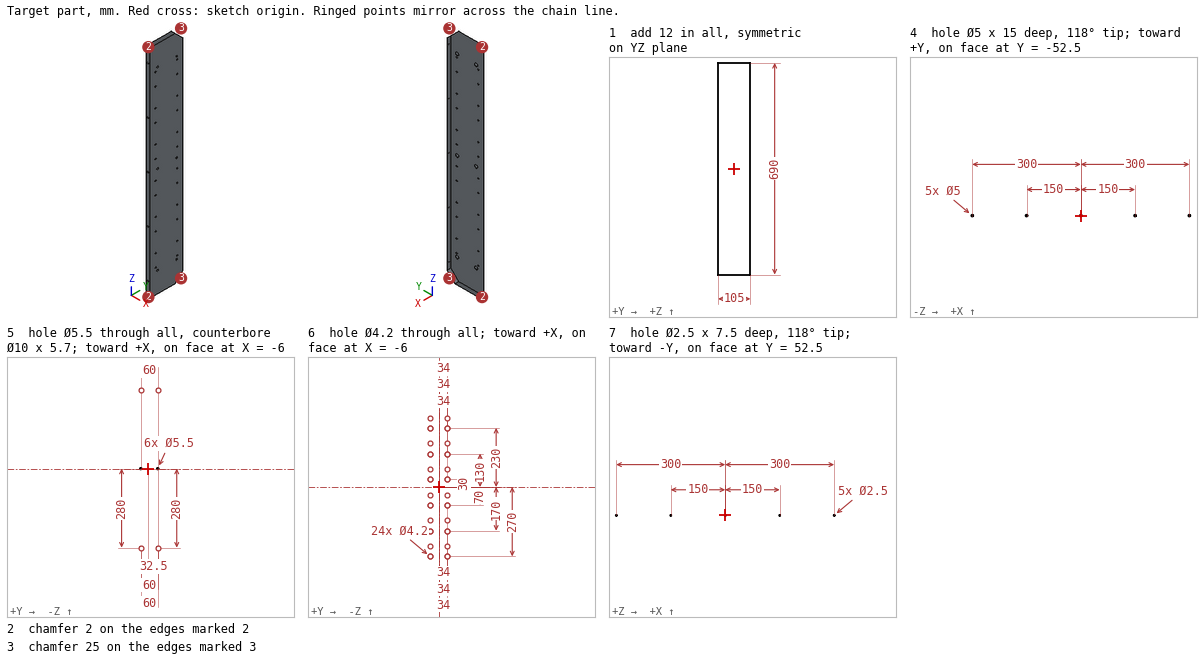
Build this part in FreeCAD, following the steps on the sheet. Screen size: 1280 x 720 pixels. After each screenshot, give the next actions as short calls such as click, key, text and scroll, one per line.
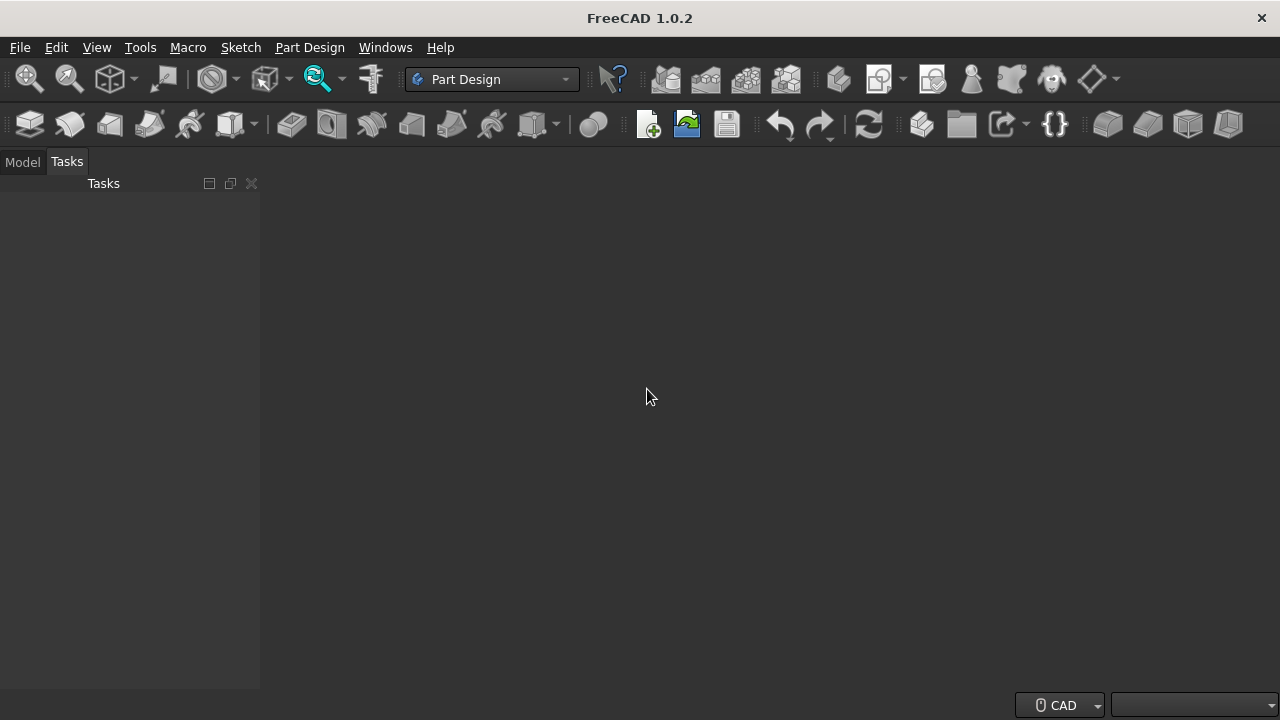
key(ctrl+n)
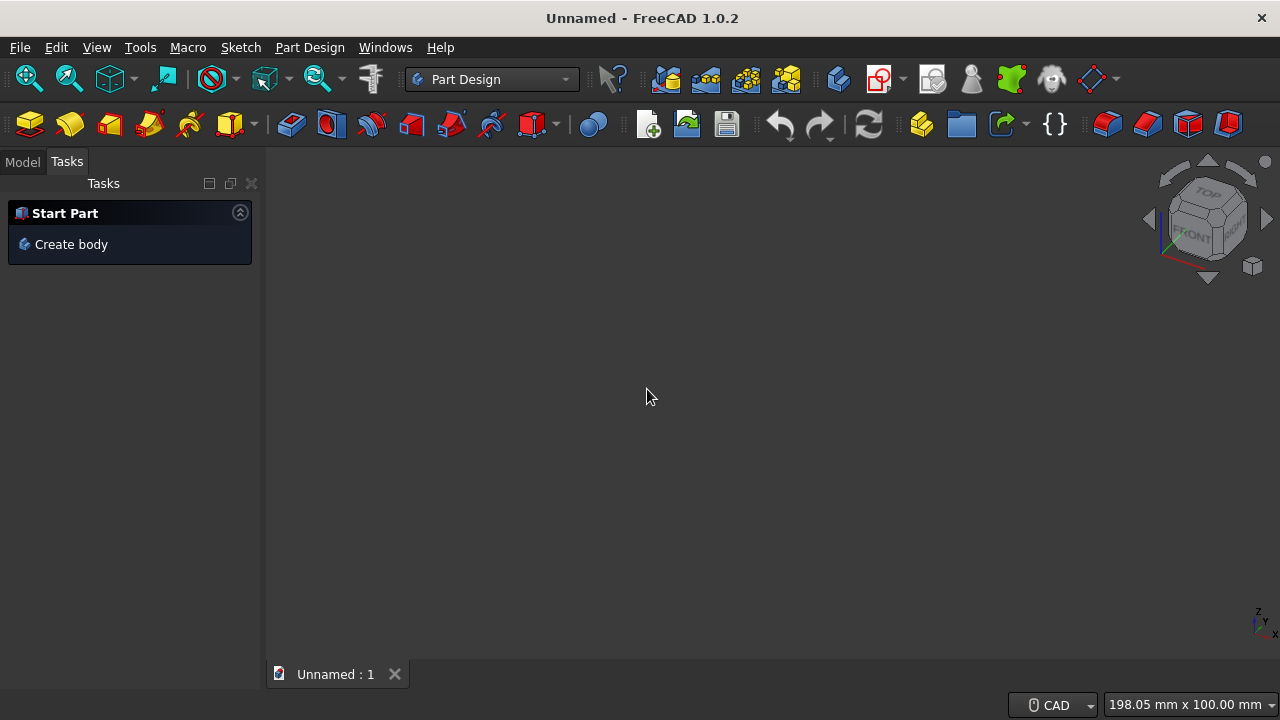
click(880, 80)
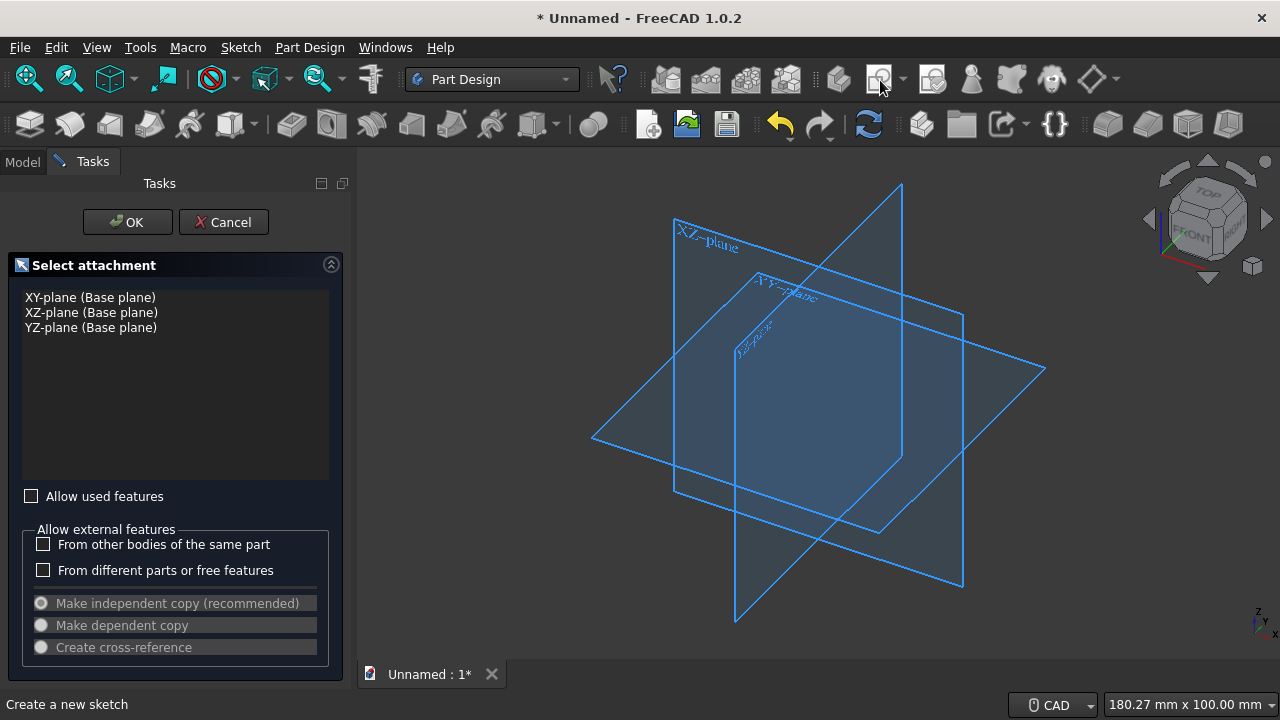
click(82, 328)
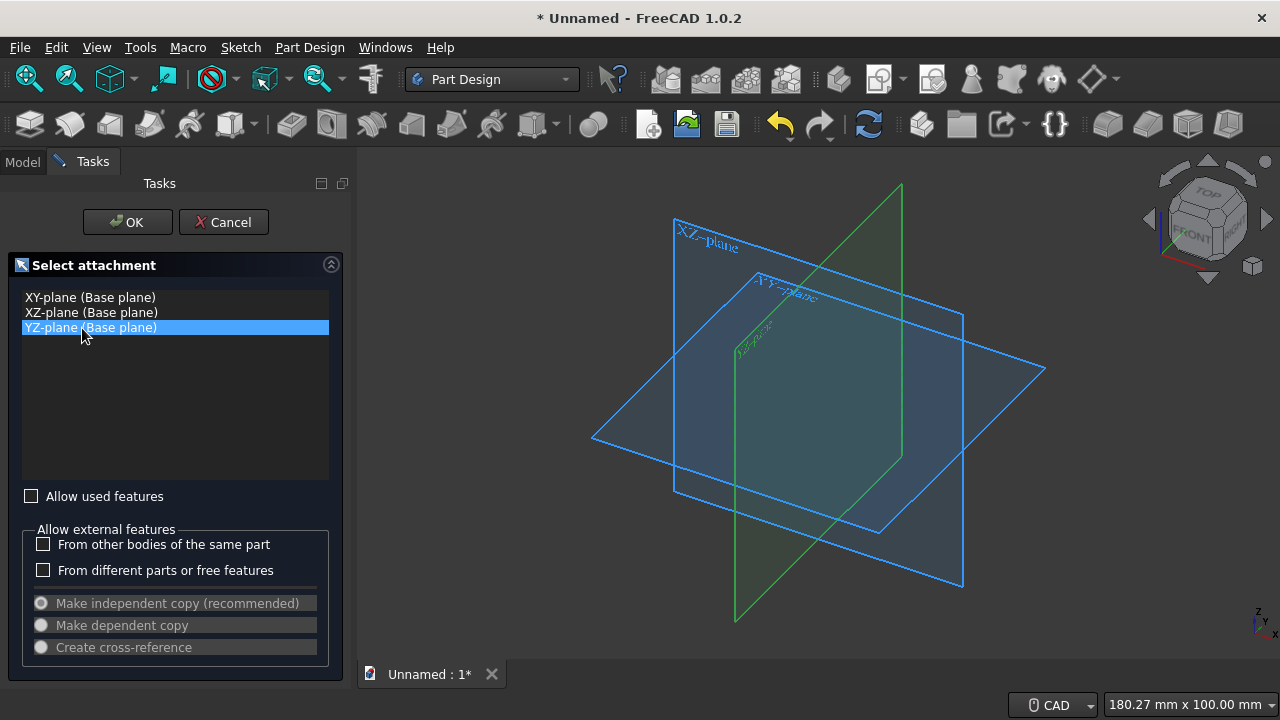
click(128, 222)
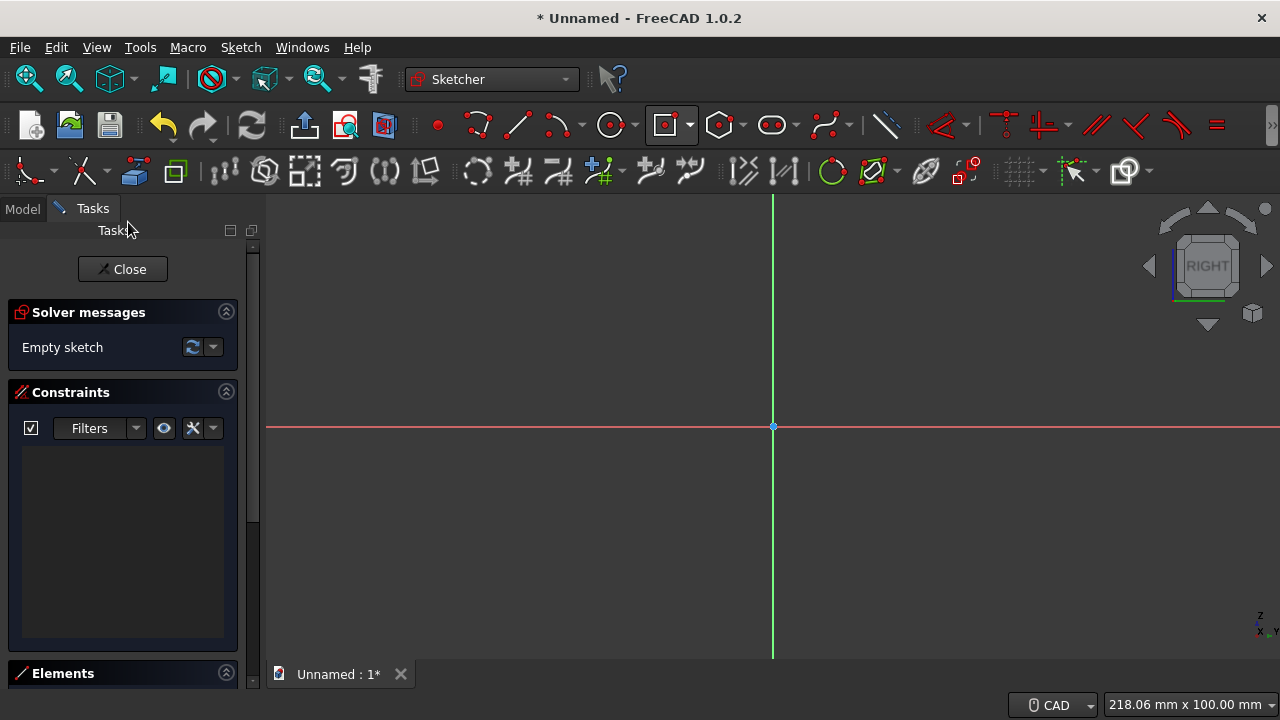
scroll(698, 426, down, 12)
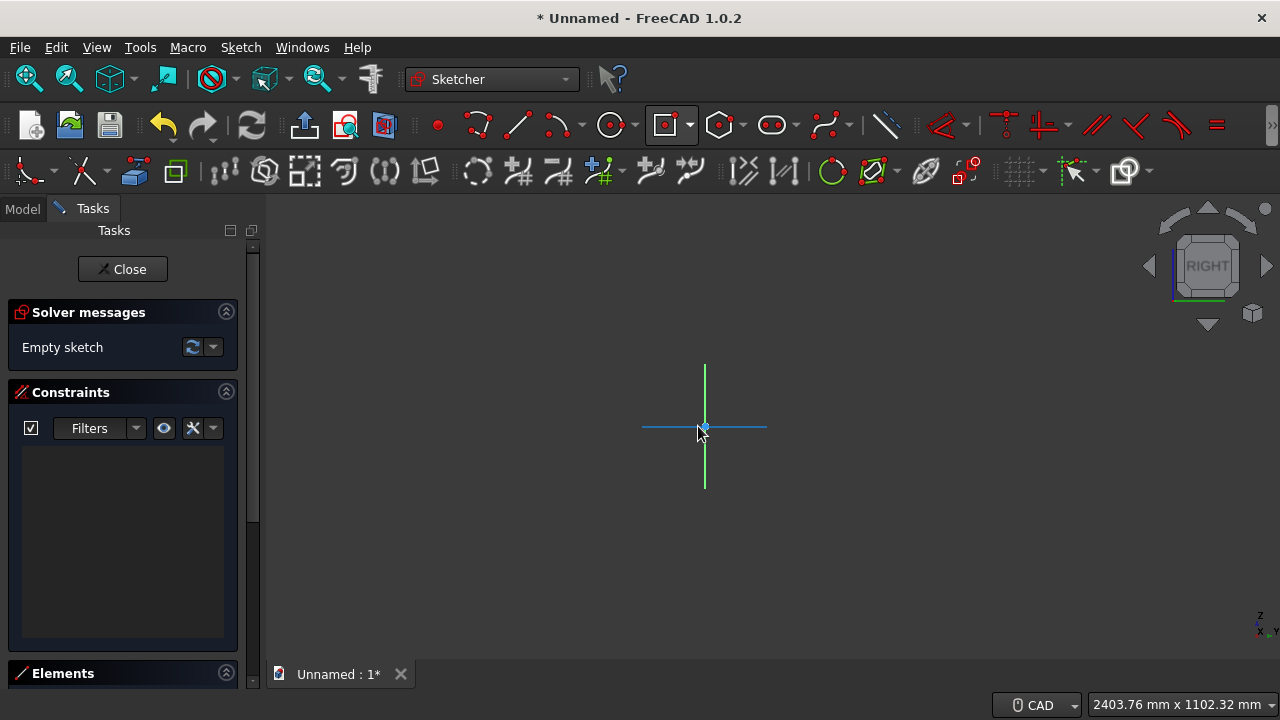
click(666, 126)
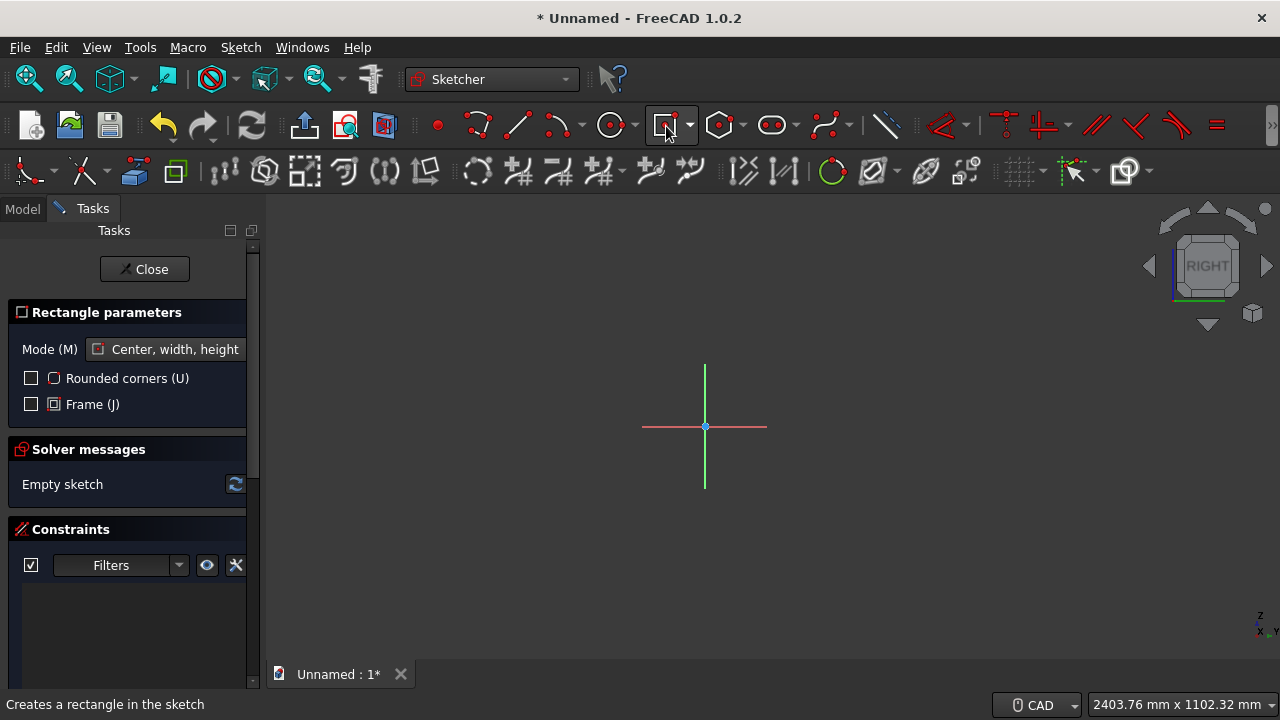
click(705, 426)
move(727, 281)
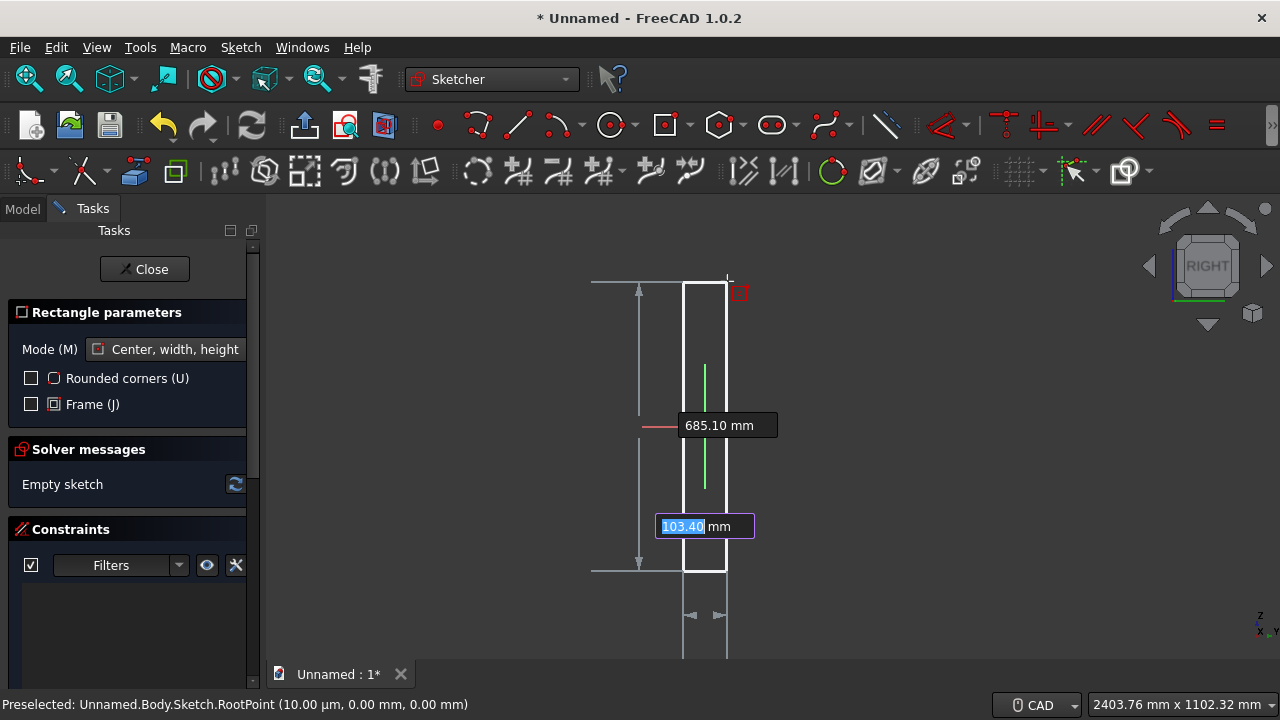
text(105)
key(Tab)
text(690)
key(Return)
key(Escape)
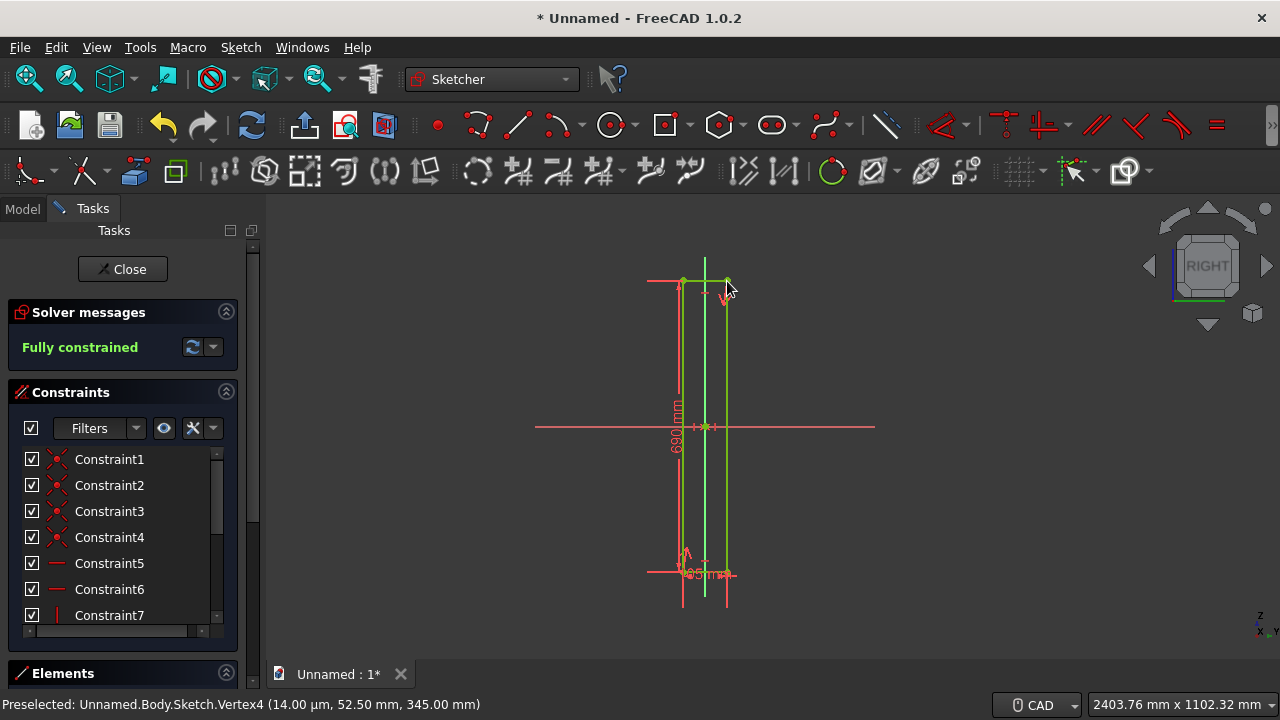
click(123, 269)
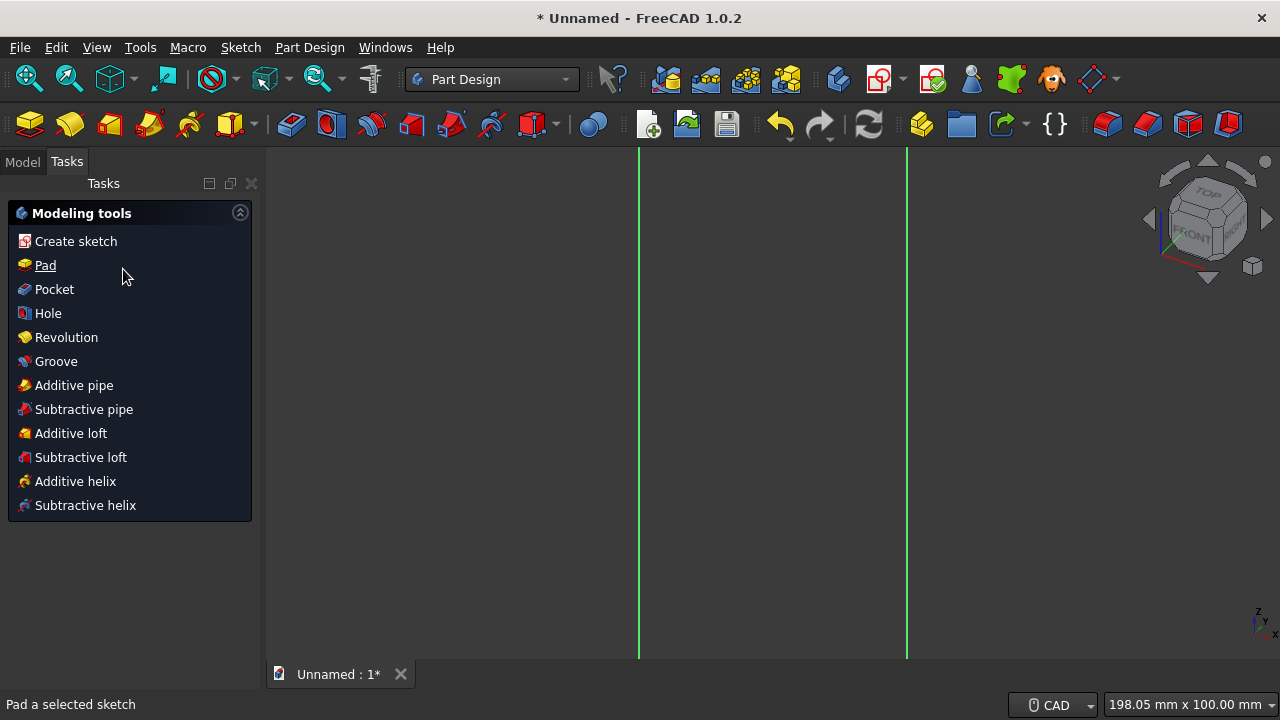
click(30, 124)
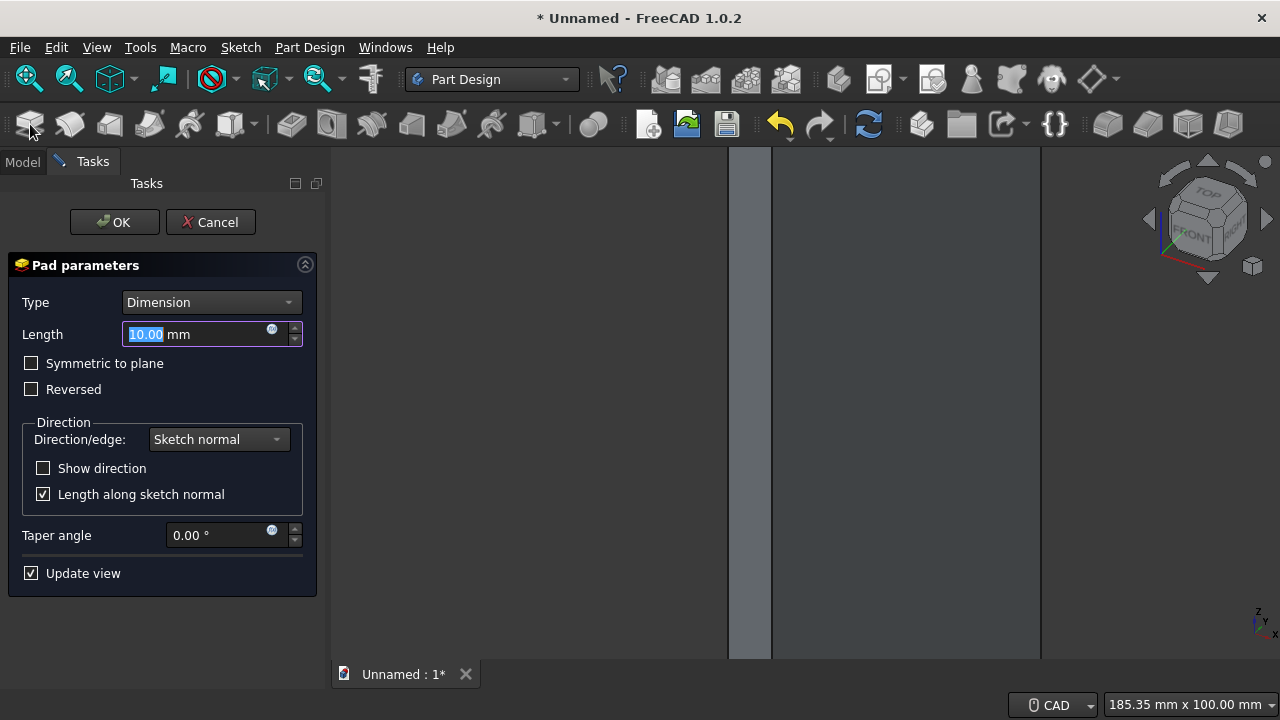
text(12)
key(Tab)